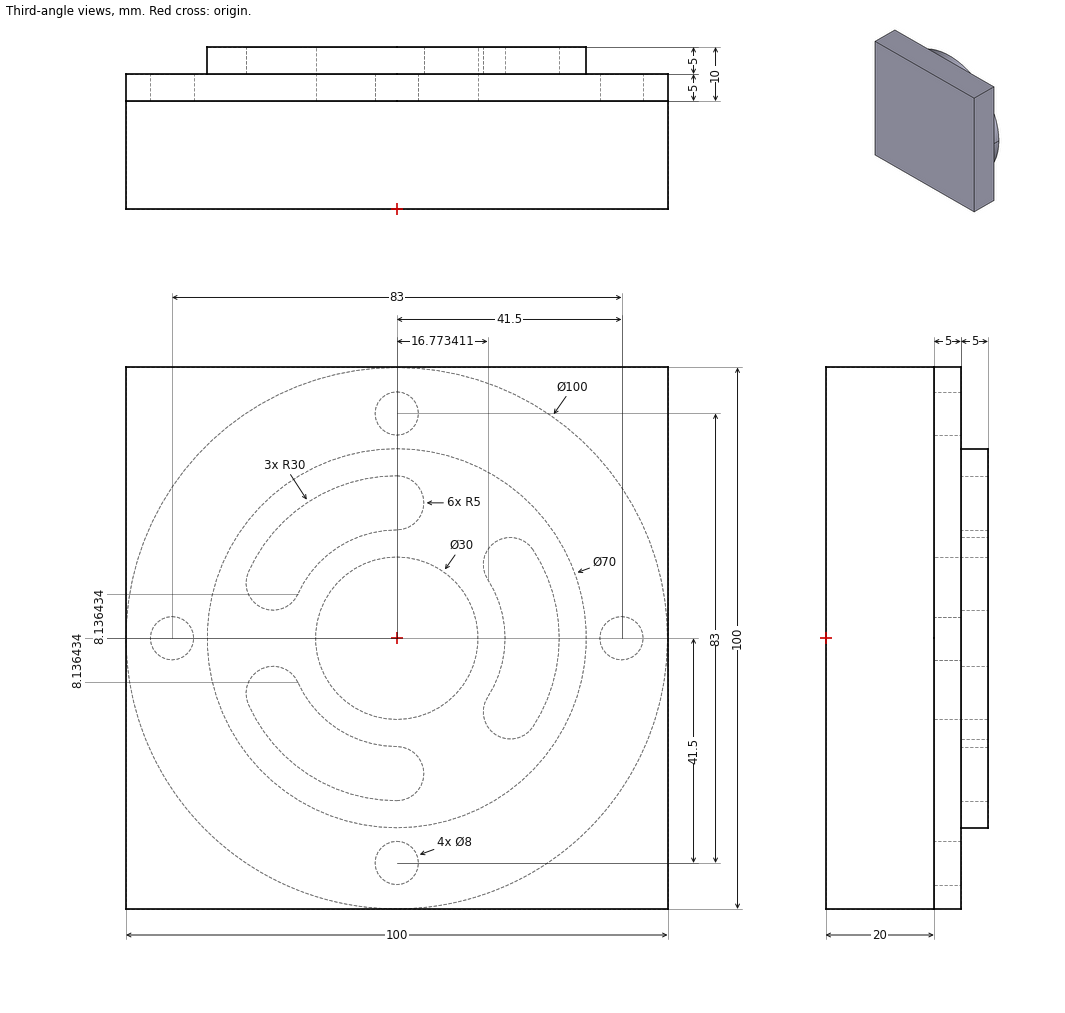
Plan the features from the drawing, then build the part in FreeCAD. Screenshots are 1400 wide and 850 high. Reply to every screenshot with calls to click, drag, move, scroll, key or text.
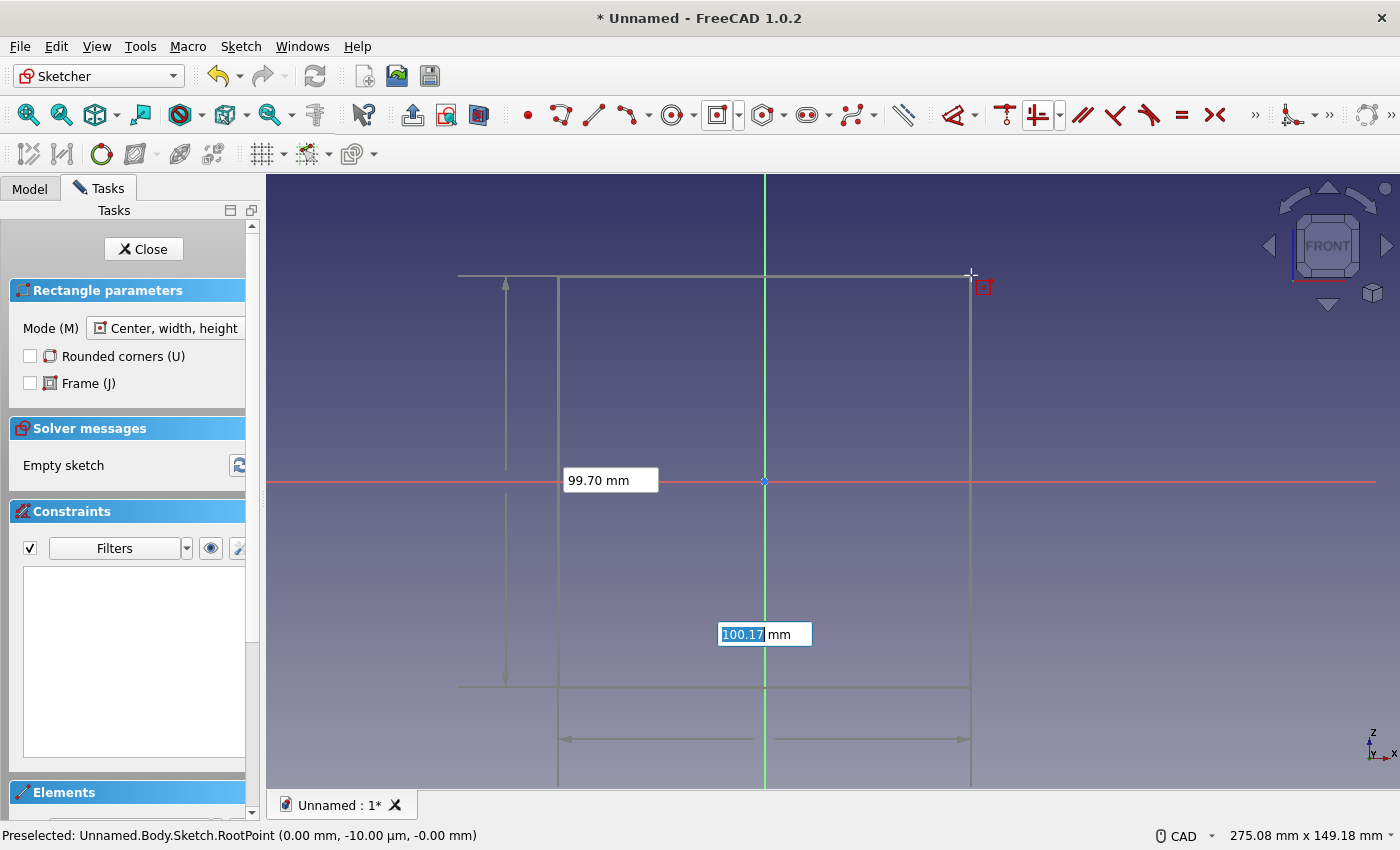
text(100)
key(Tab)
text(100)
key(Return)
key(Escape)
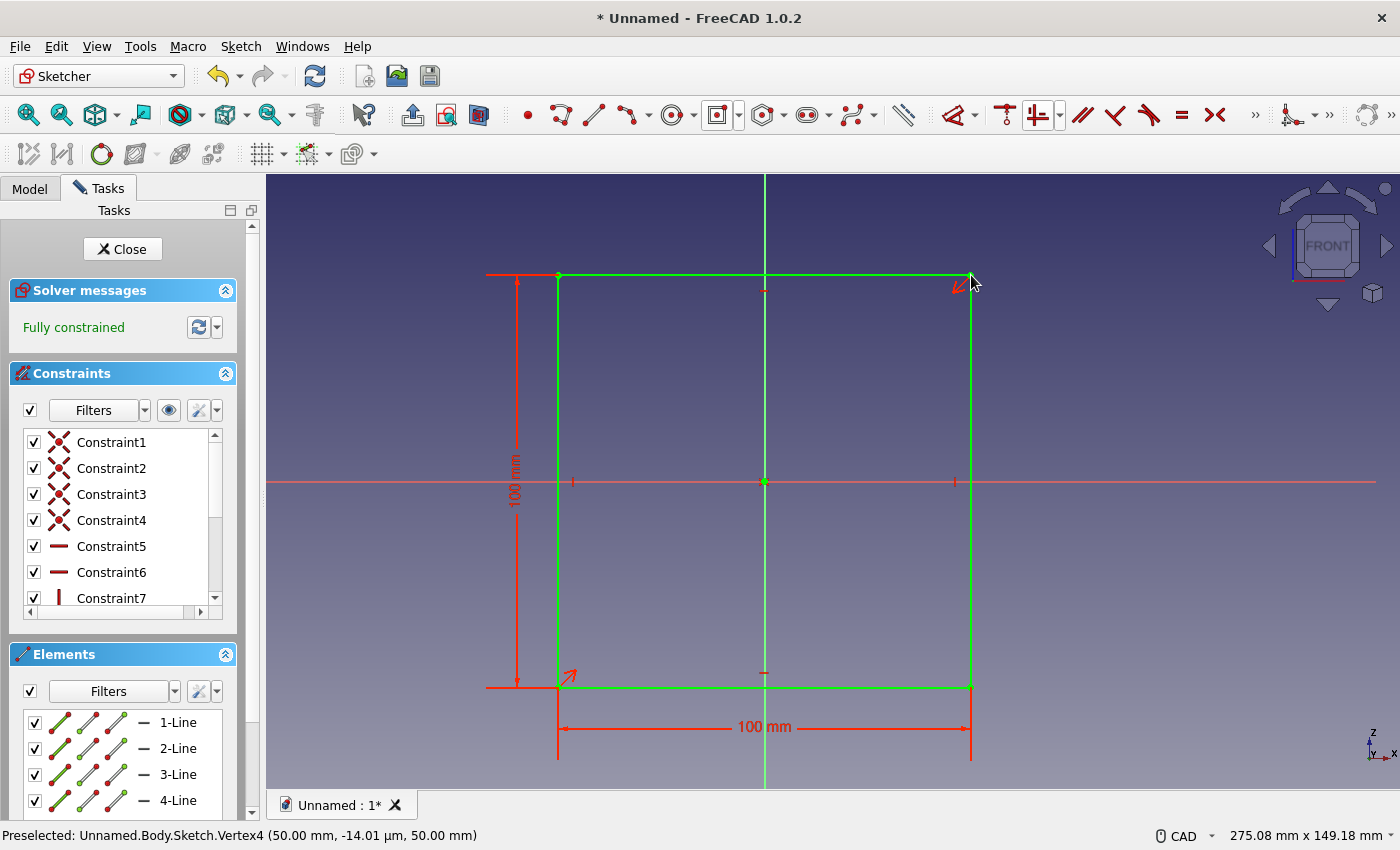
click(123, 249)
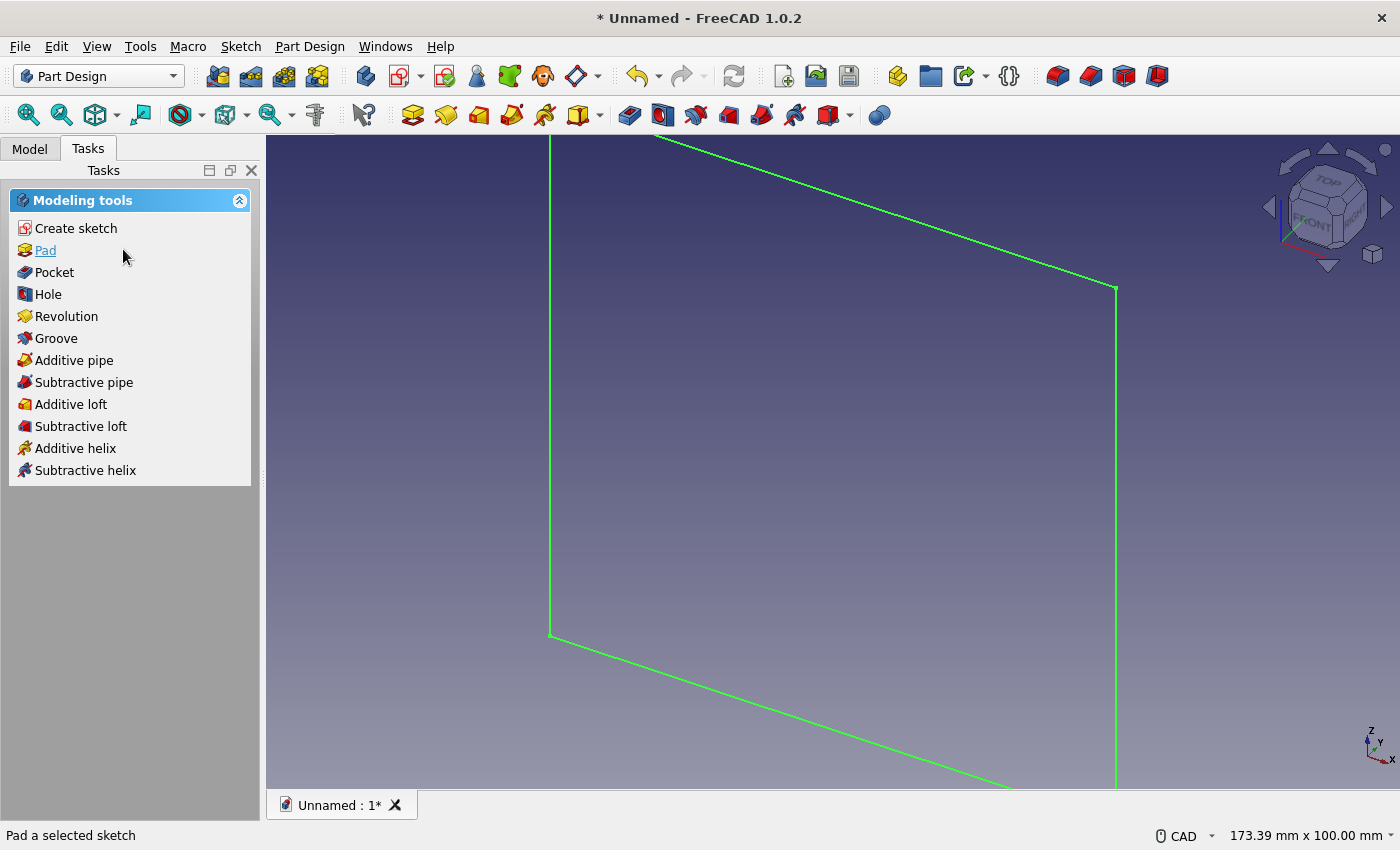
click(413, 116)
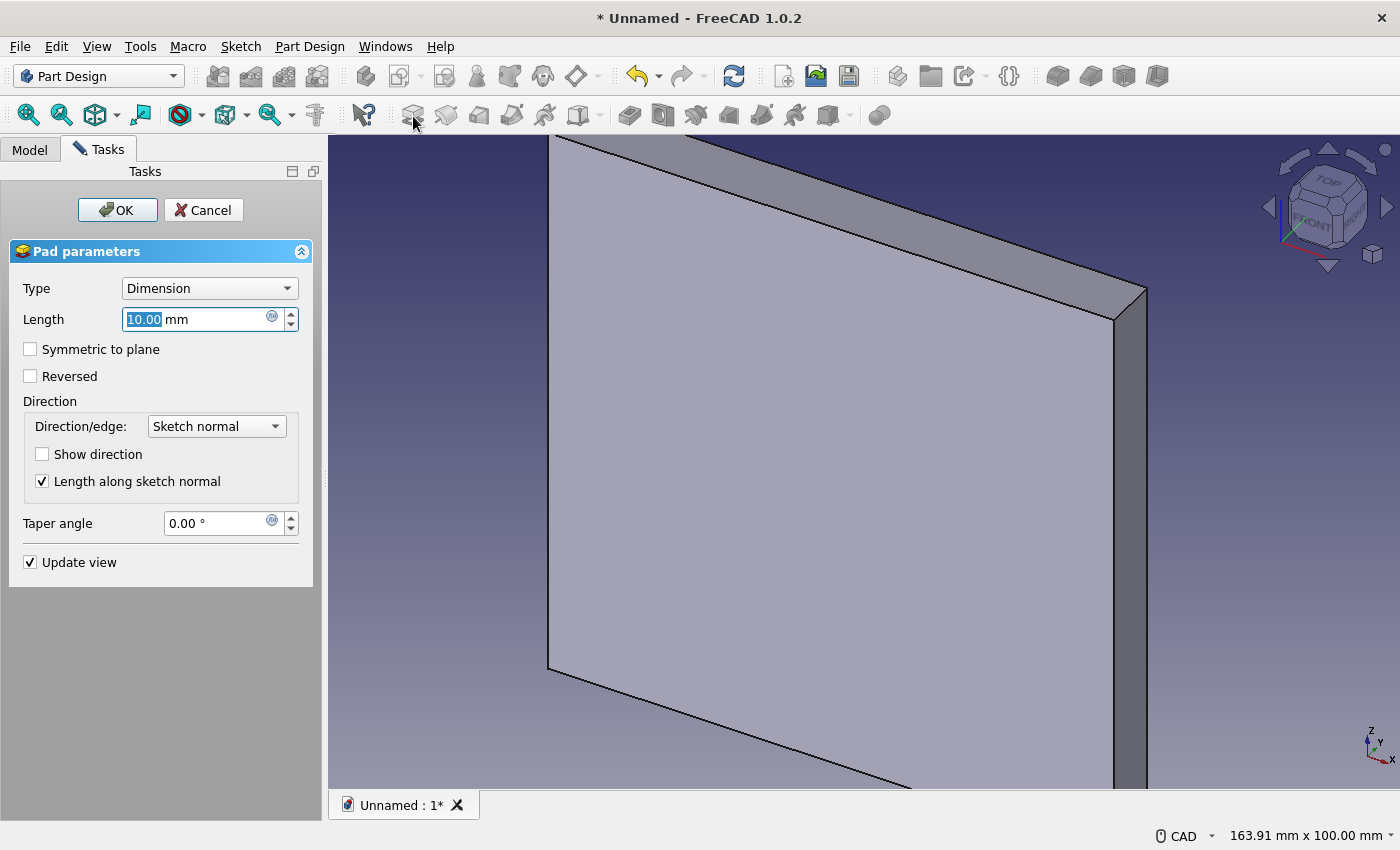
text(20)
key(Tab)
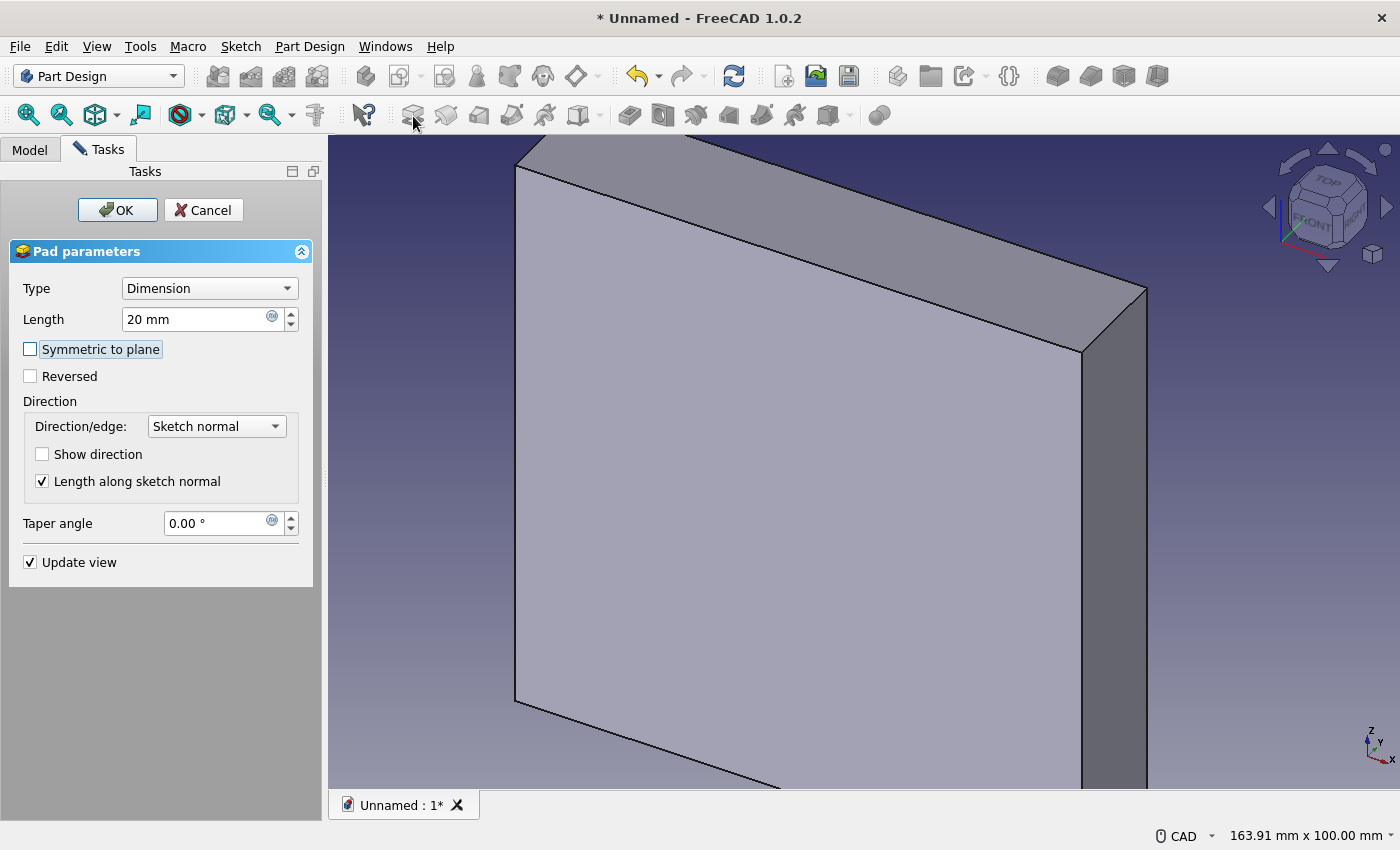
click(31, 376)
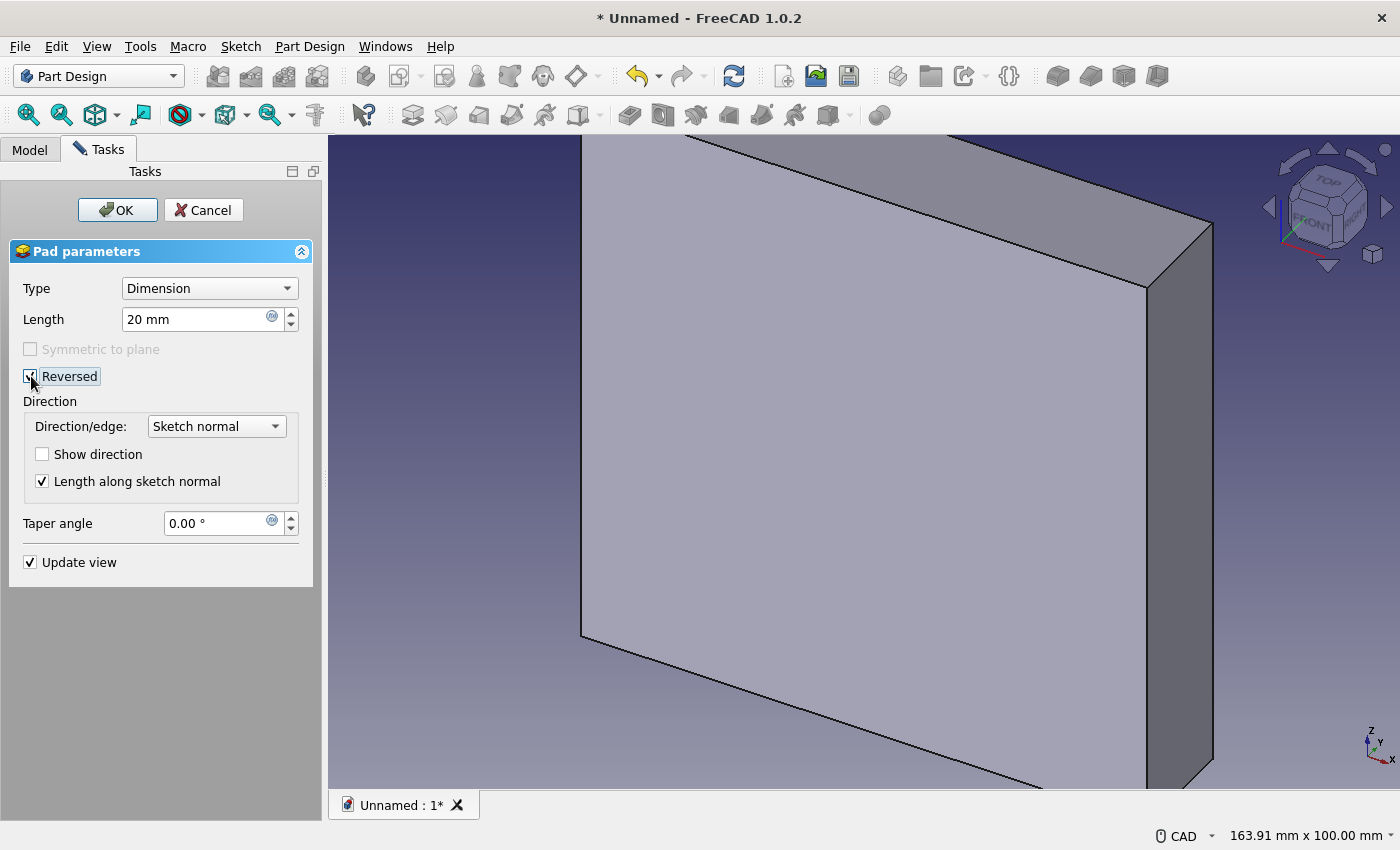
click(118, 210)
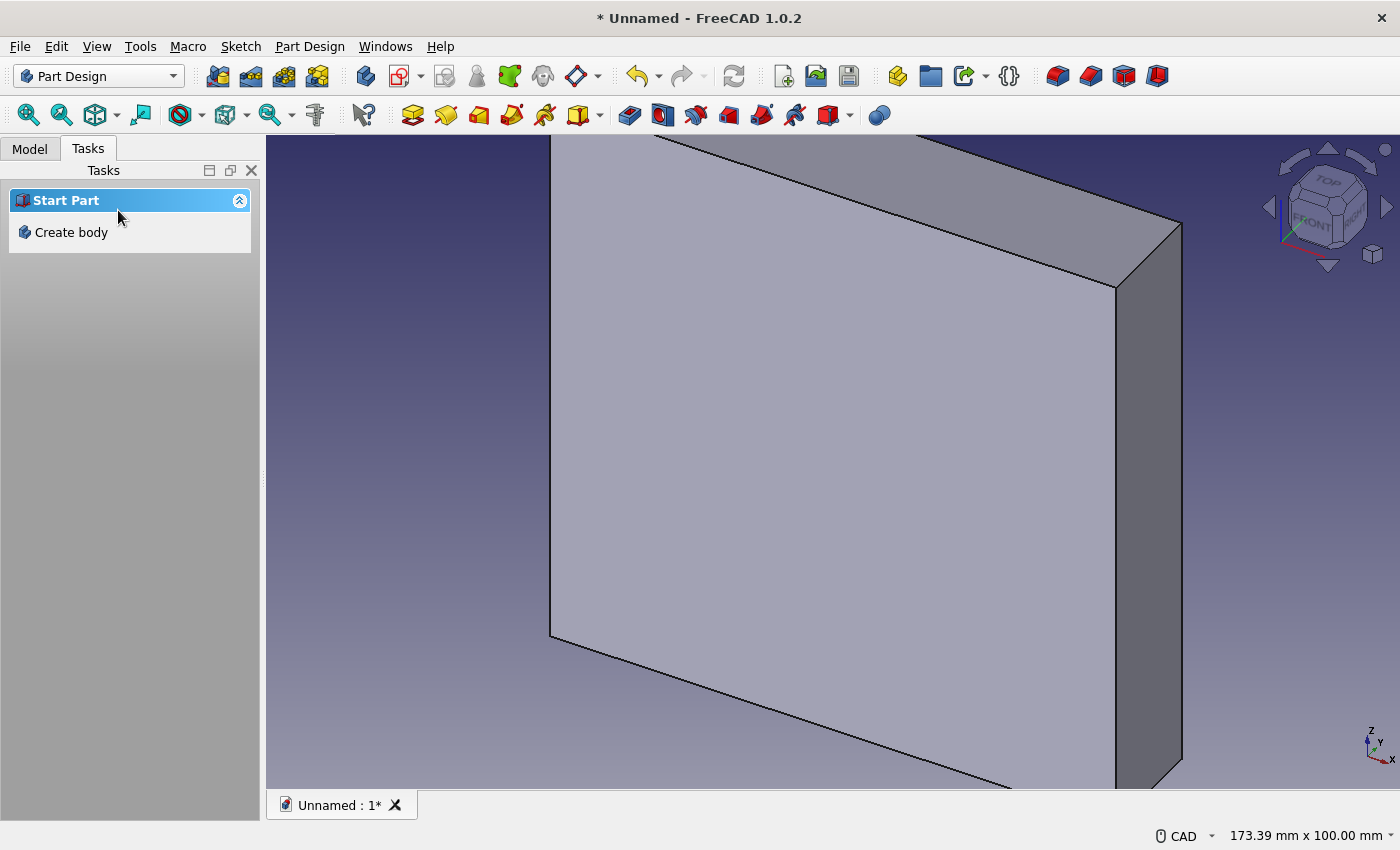
click(29, 116)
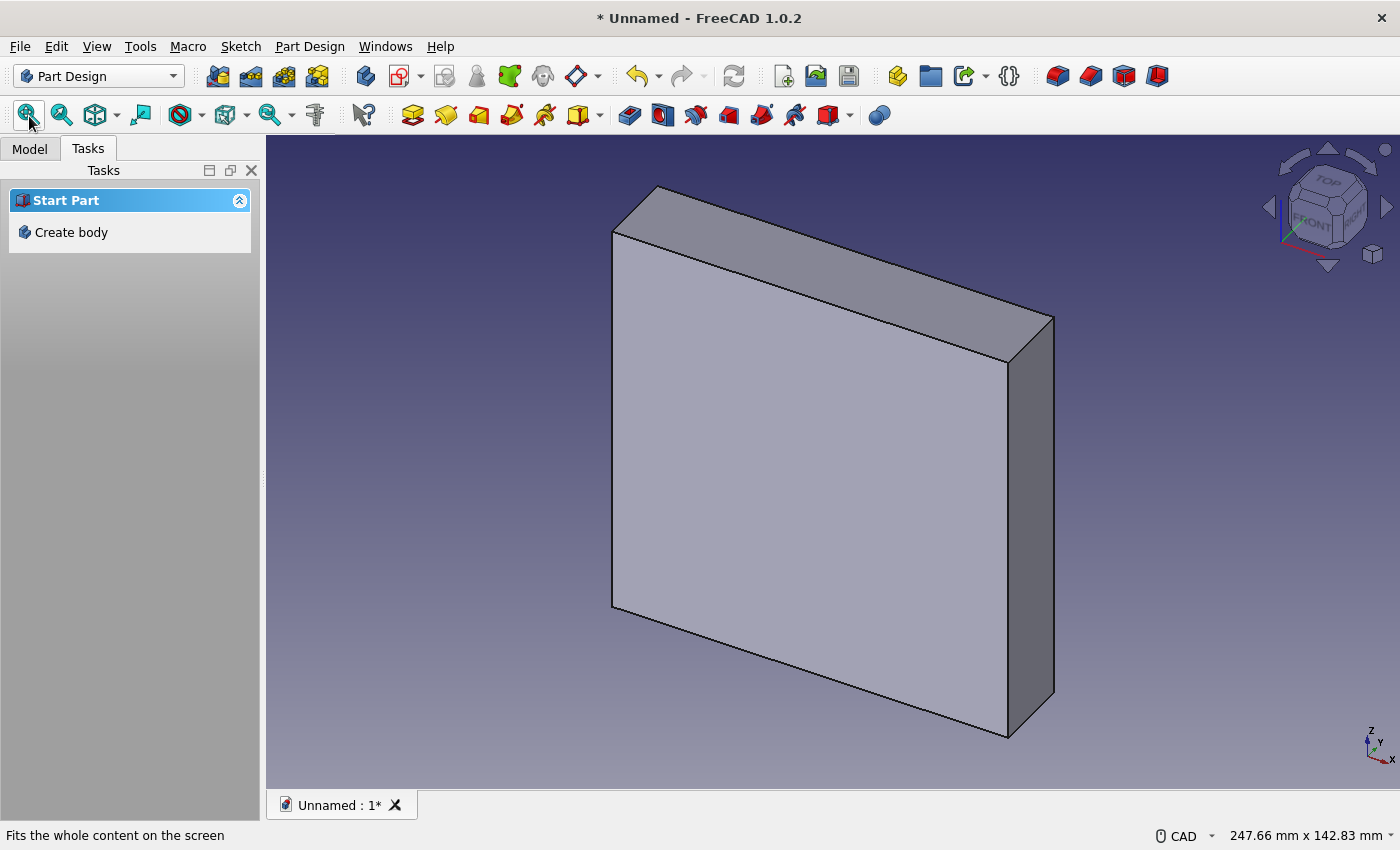
key(4)